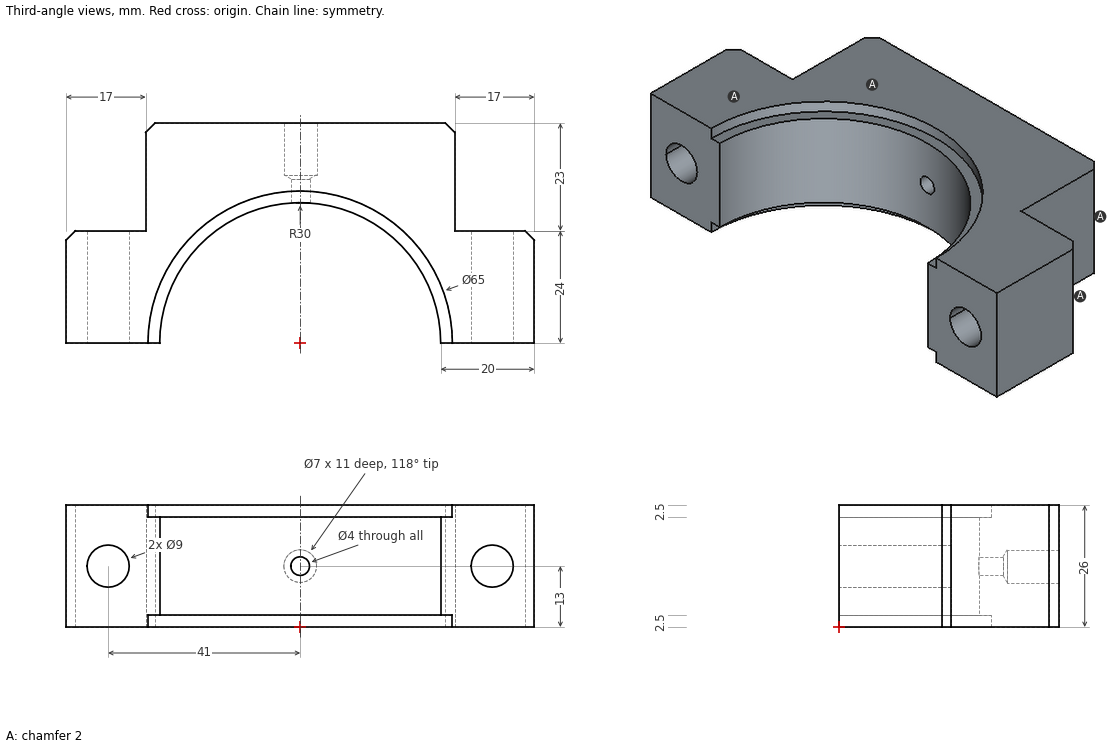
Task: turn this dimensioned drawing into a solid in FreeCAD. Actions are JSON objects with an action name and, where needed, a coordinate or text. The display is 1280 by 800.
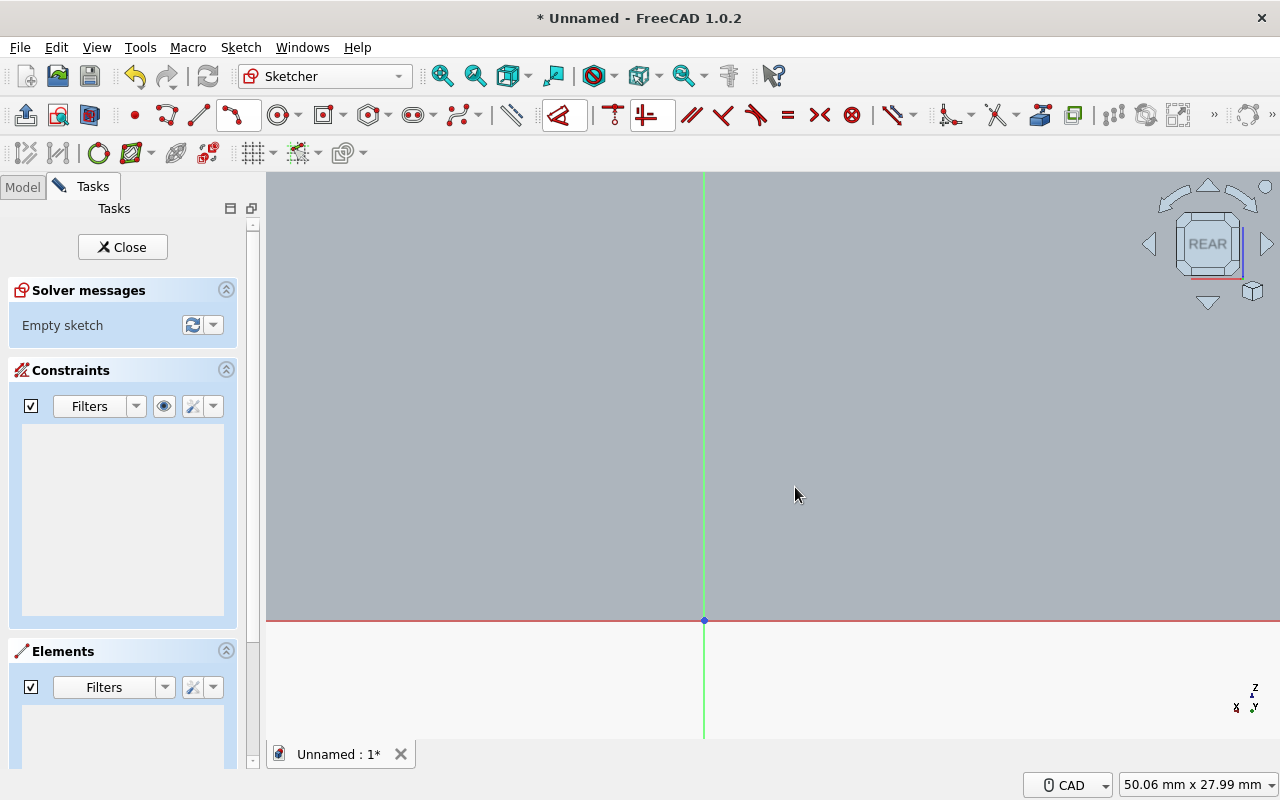
{"action": "key", "text": "g c"}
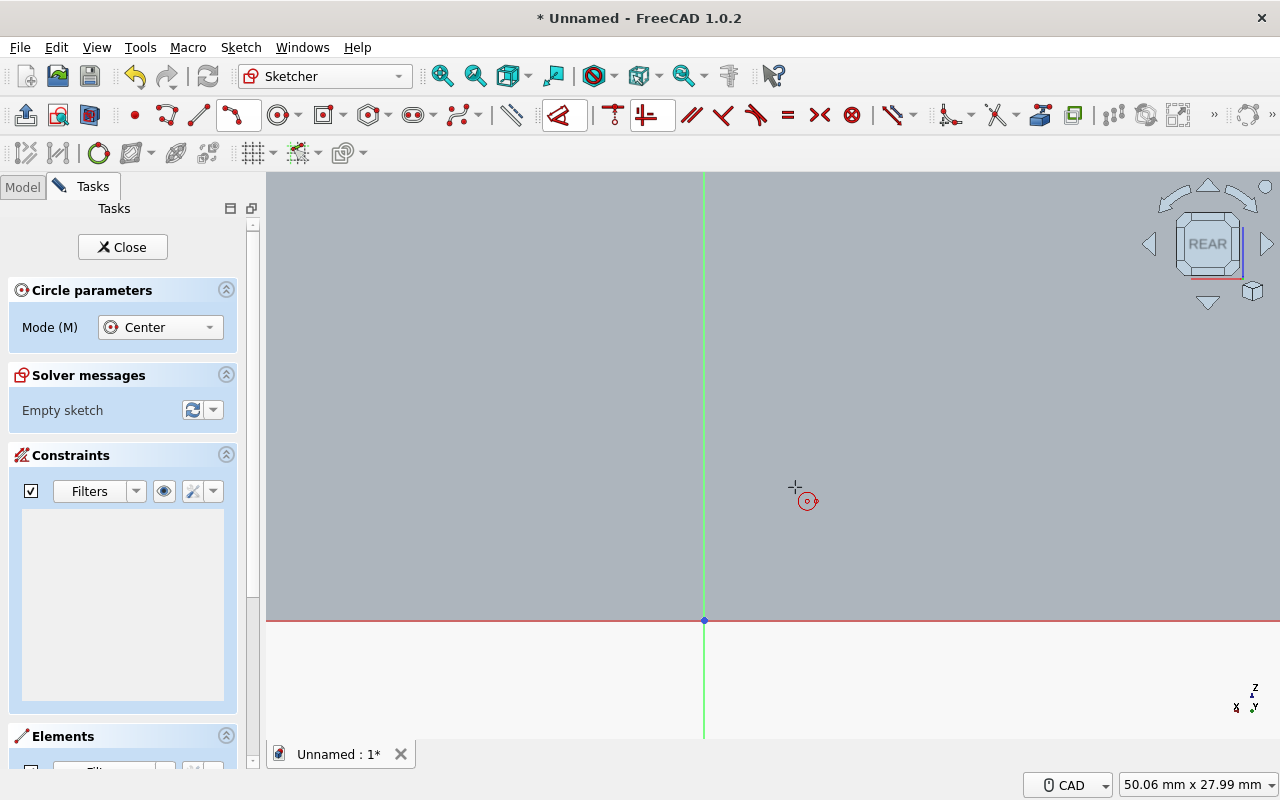
{"action": "left_click", "coordinate": [704, 358]}
{"action": "left_click", "coordinate": [754, 307]}
{"action": "key", "text": "Escape"}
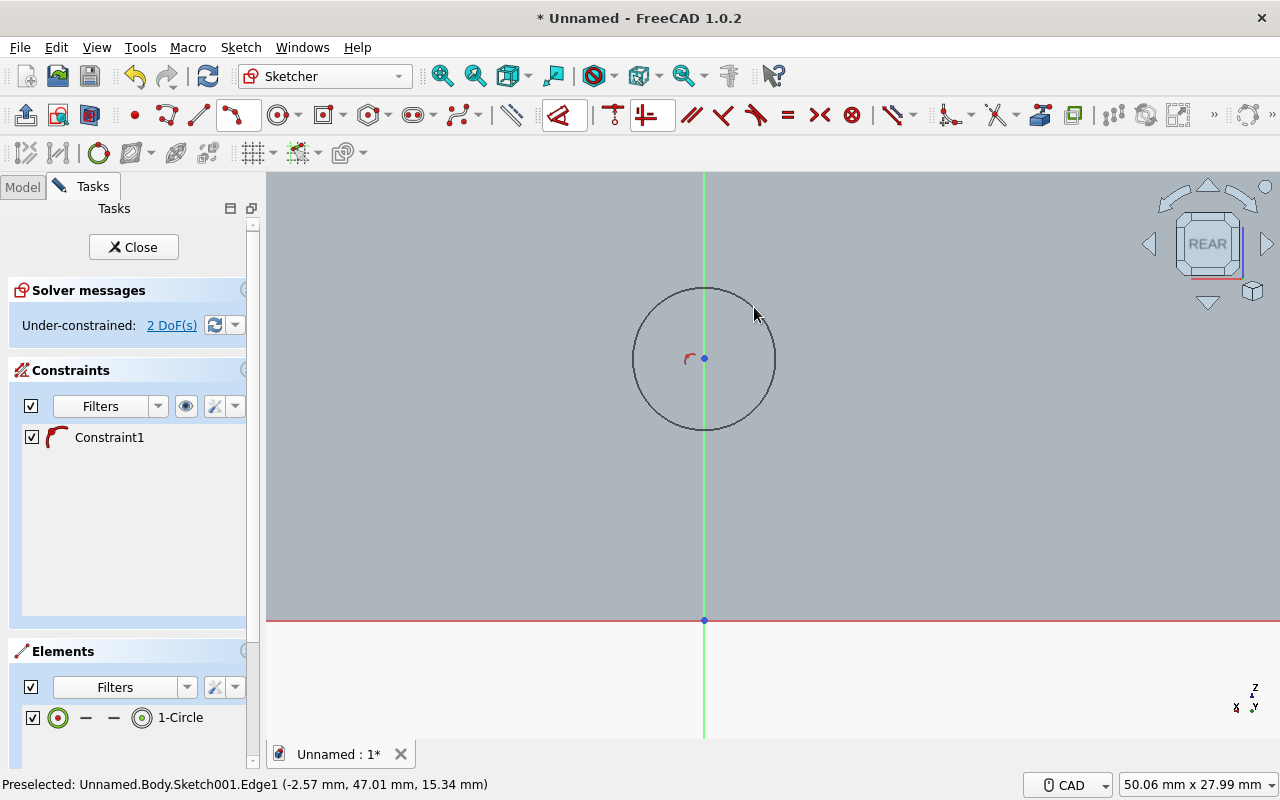
{"action": "left_click", "coordinate": [754, 308]}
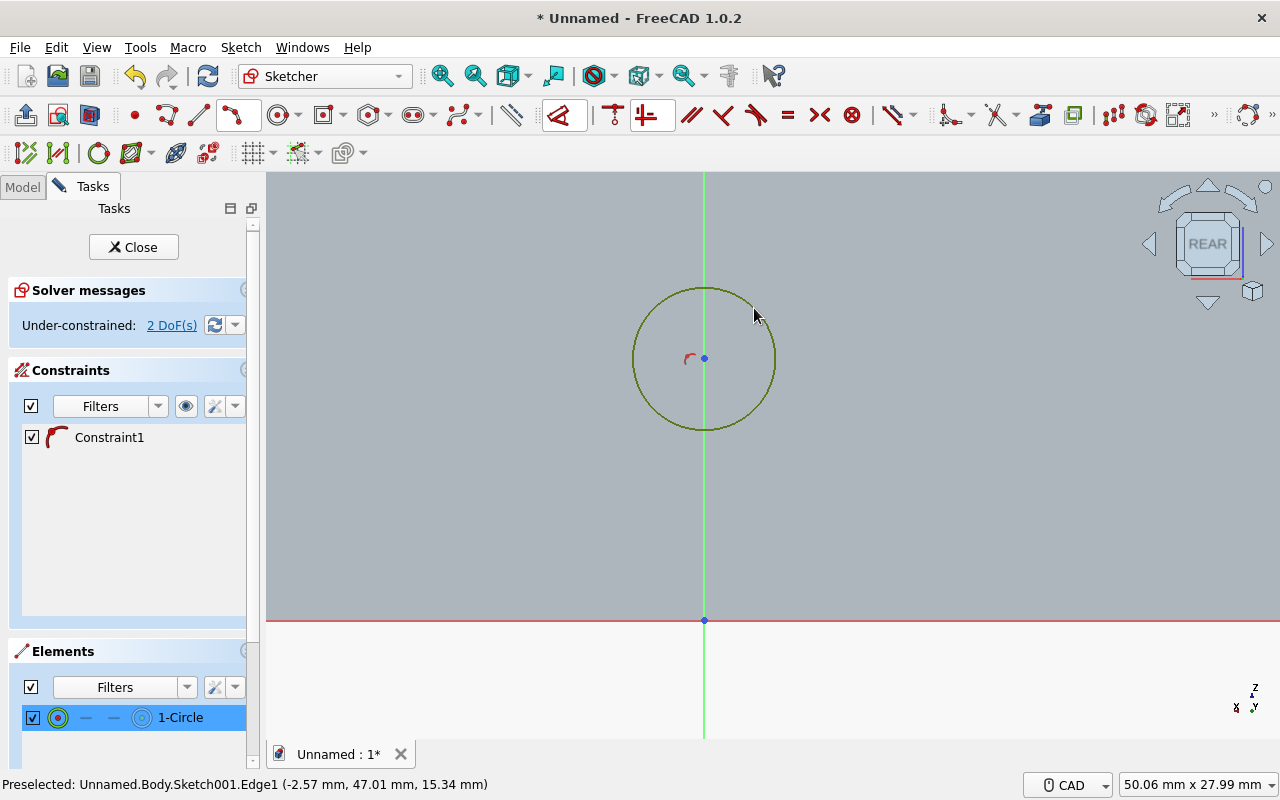
{"action": "key", "text": "k o"}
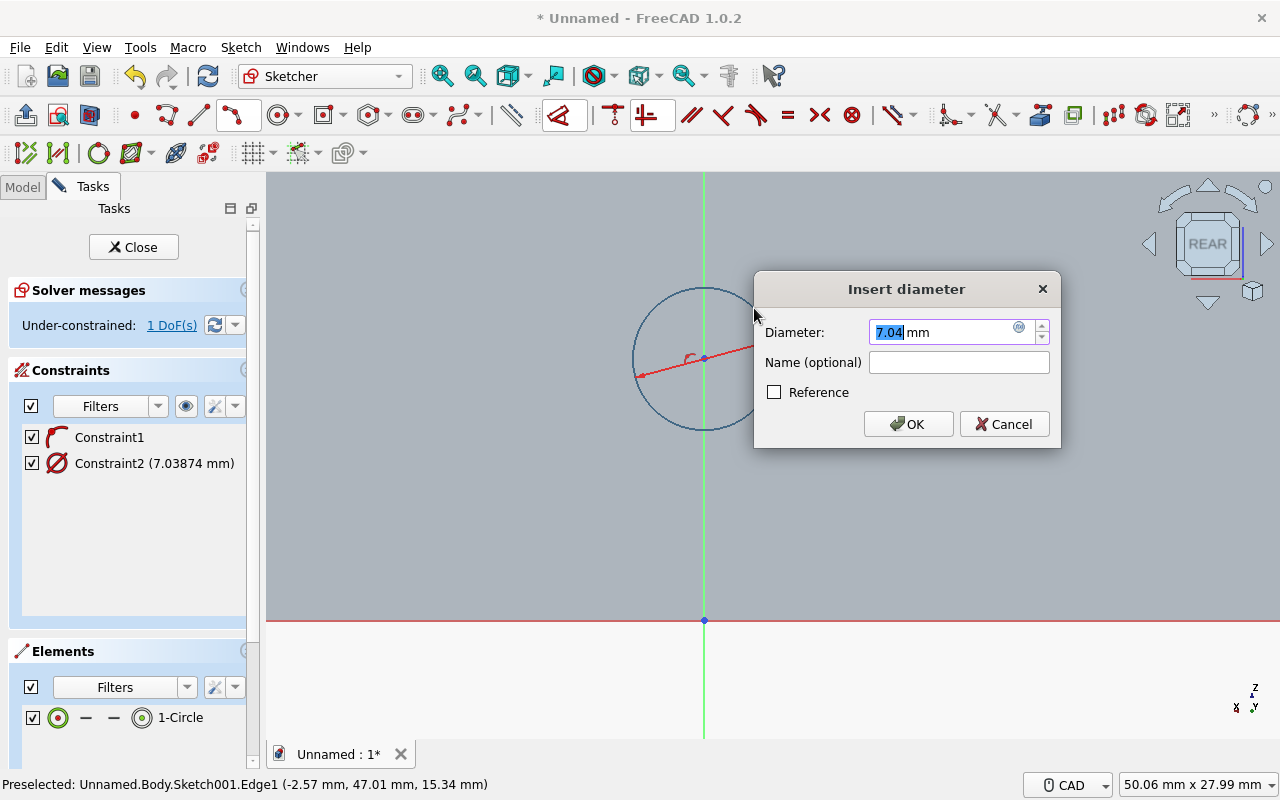
{"action": "type", "text": "7"}
{"action": "key", "text": "Return"}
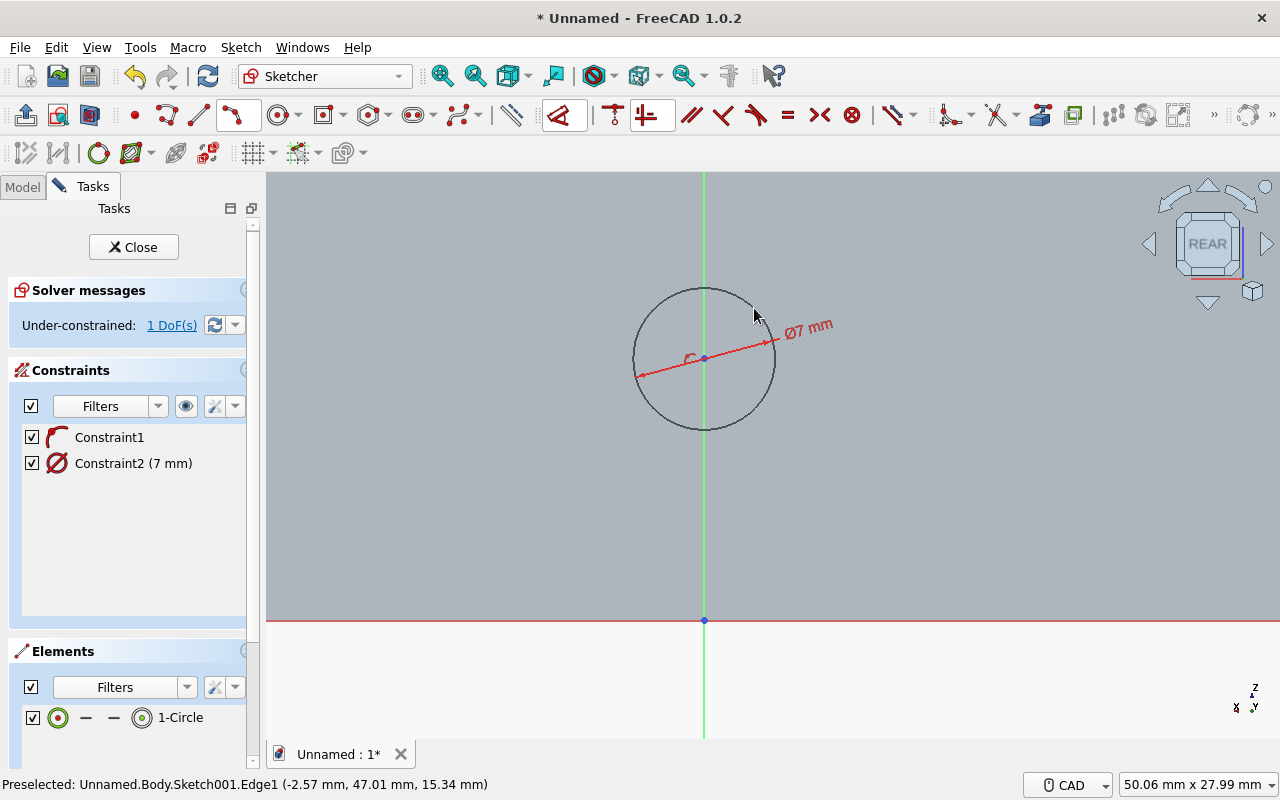
{"action": "left_click", "coordinate": [704, 359]}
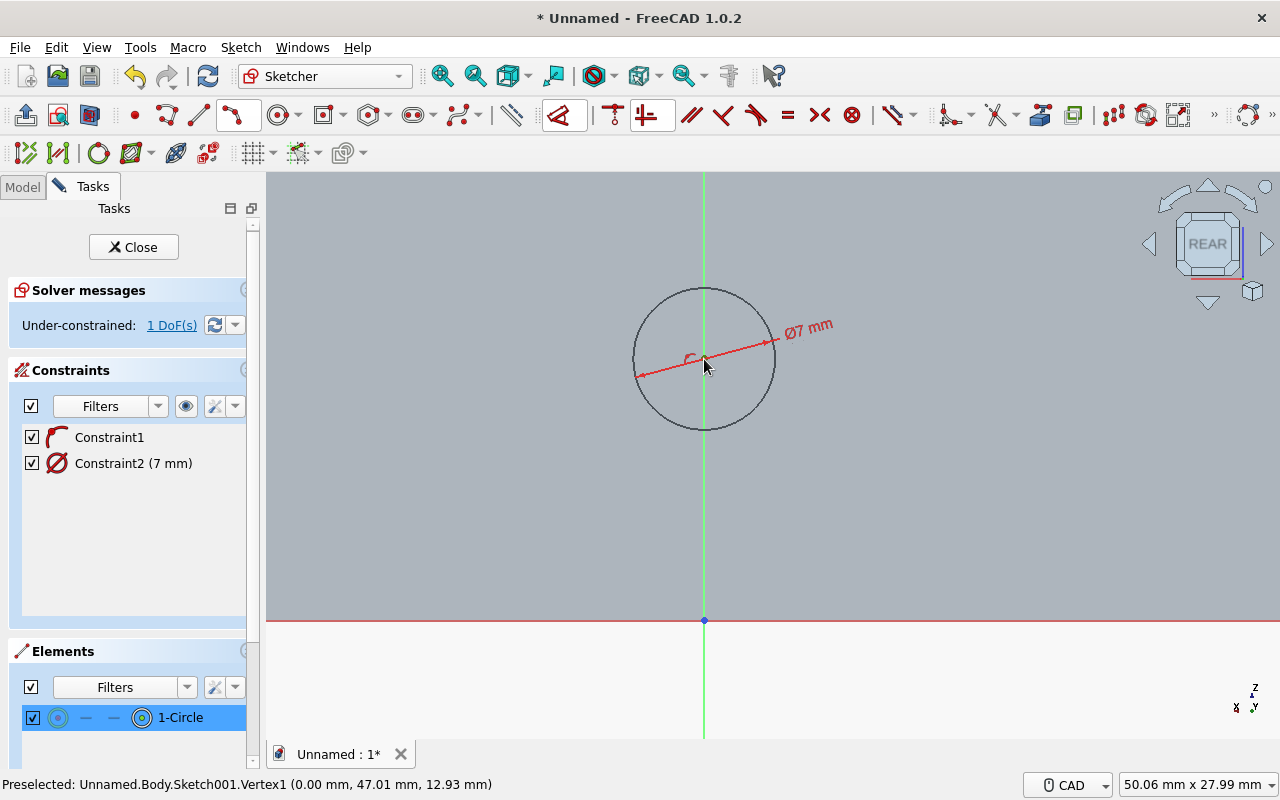
{"action": "left_click", "coordinate": [582, 116]}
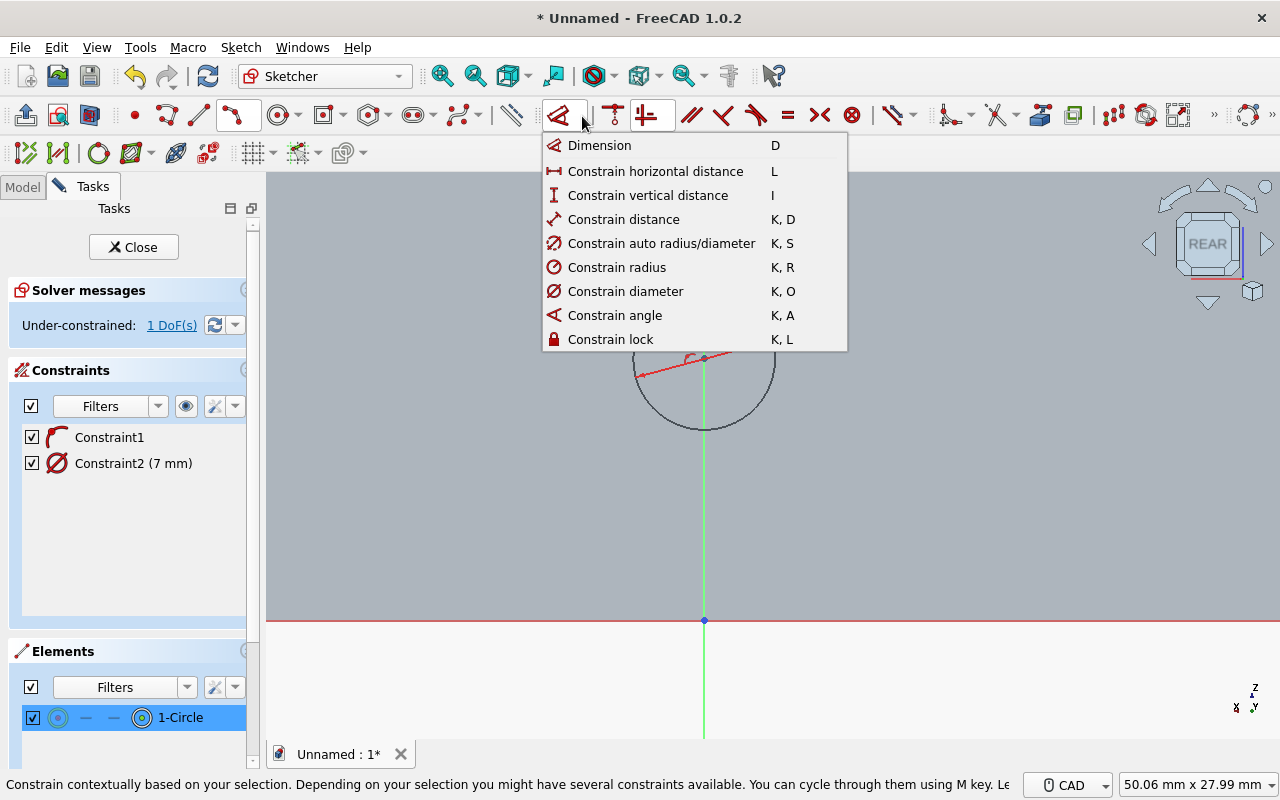
{"action": "left_click", "coordinate": [695, 195]}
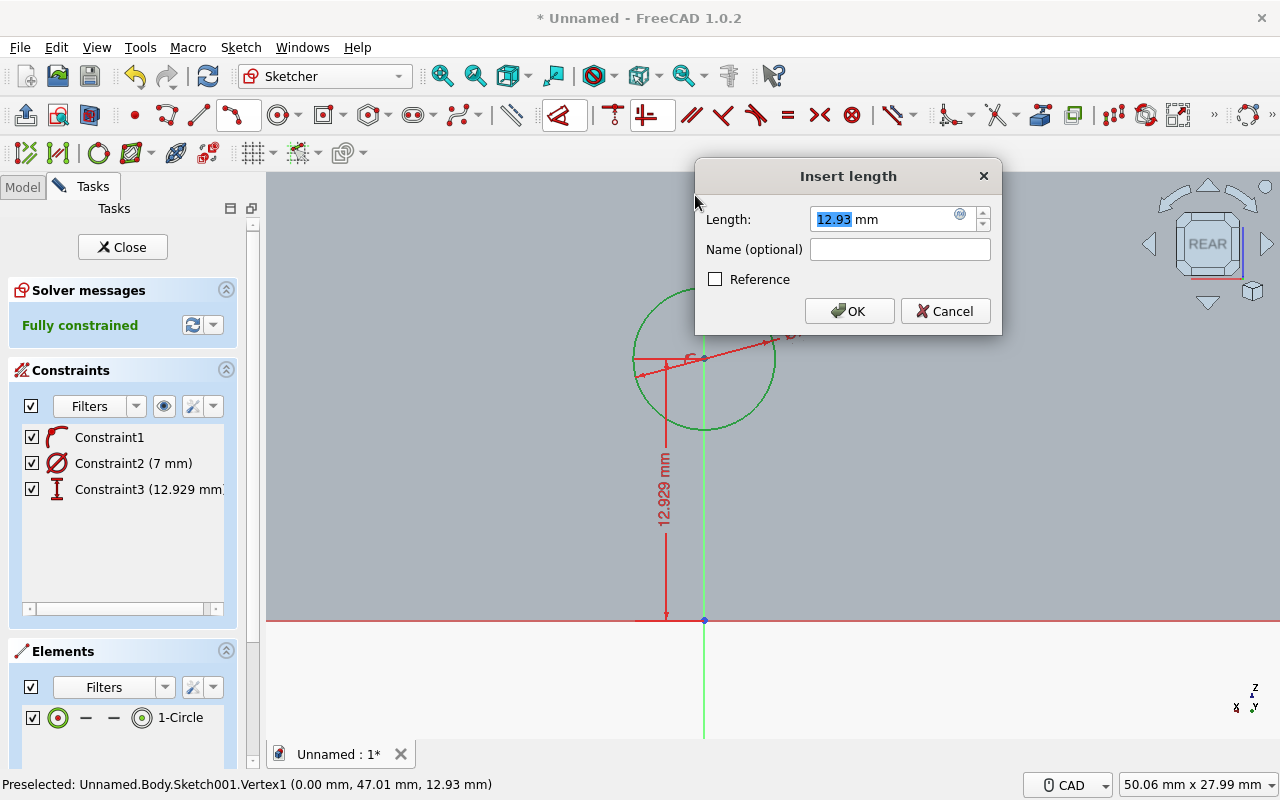
{"action": "type", "text": "13"}
{"action": "key", "text": "Return"}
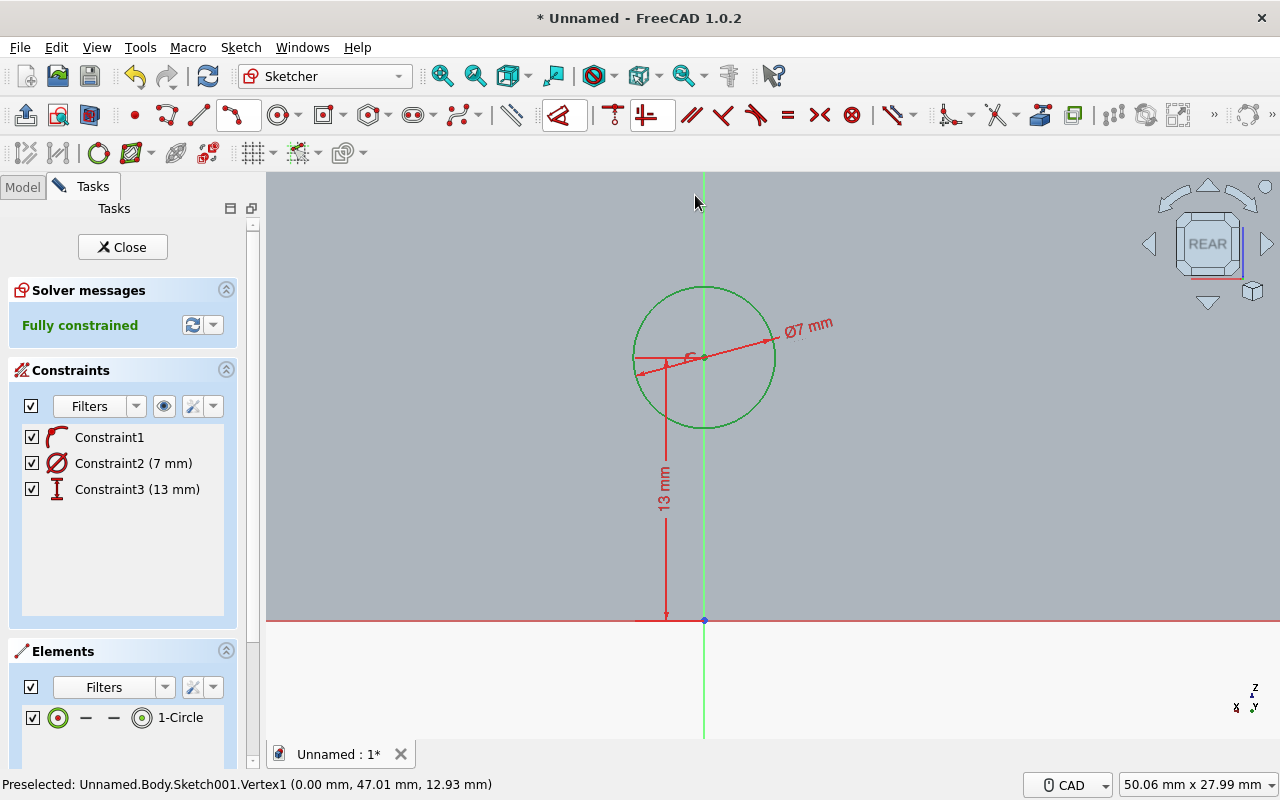
{"action": "left_click", "coordinate": [123, 247]}